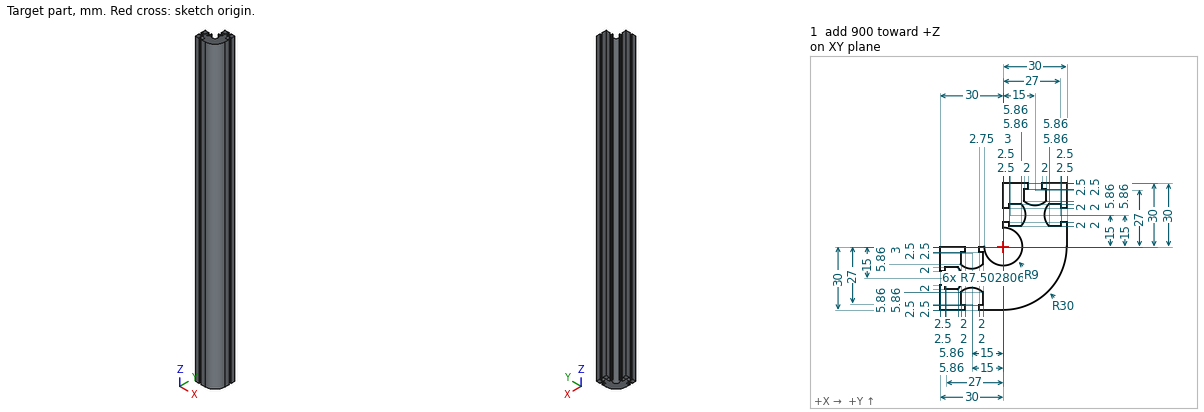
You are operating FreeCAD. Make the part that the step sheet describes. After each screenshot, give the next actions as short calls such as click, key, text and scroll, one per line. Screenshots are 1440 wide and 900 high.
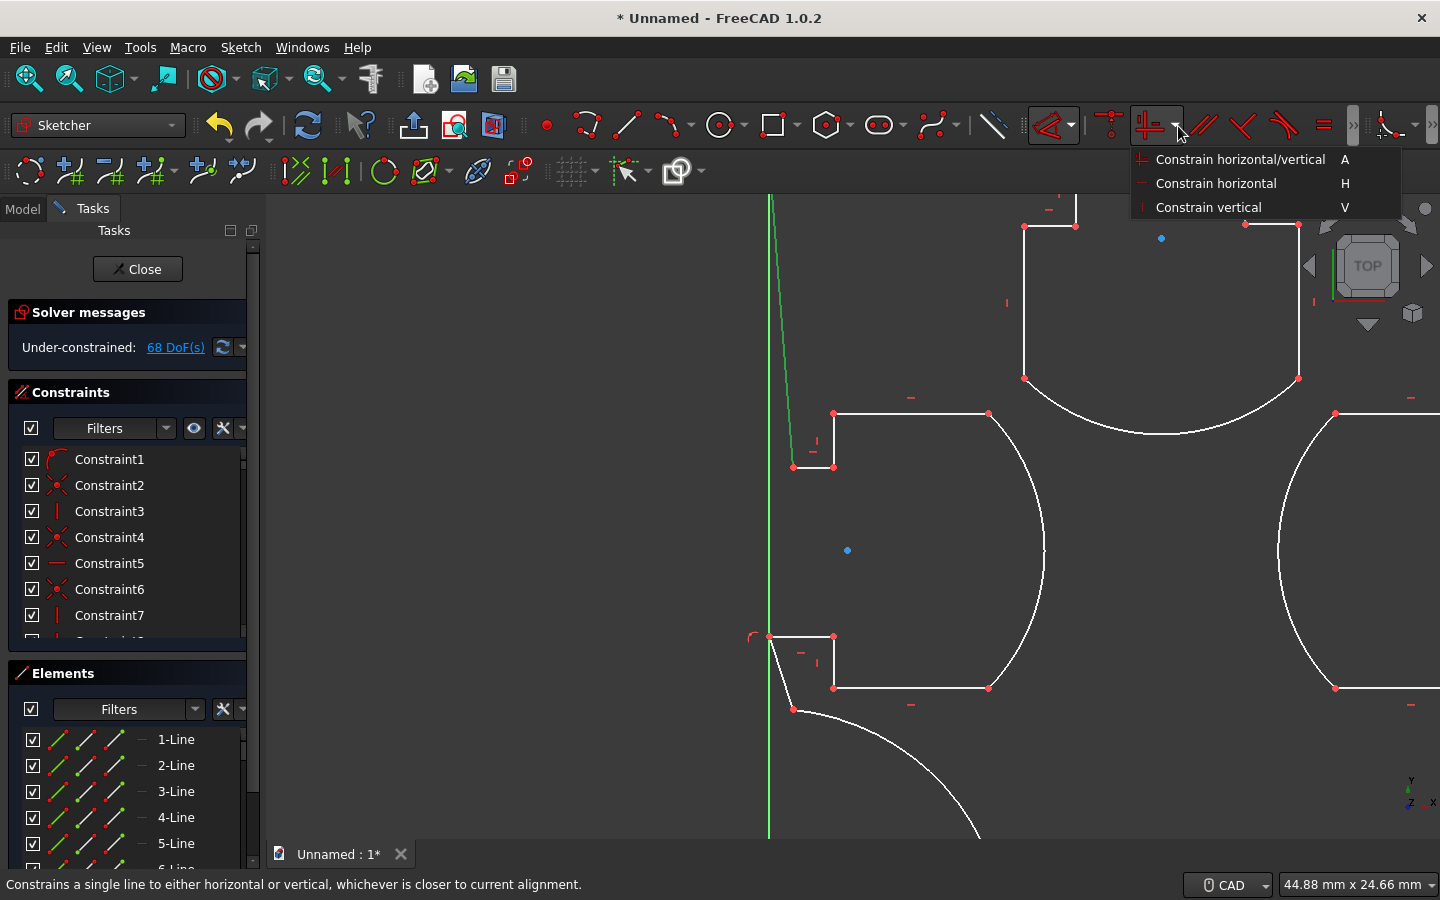
click(1266, 207)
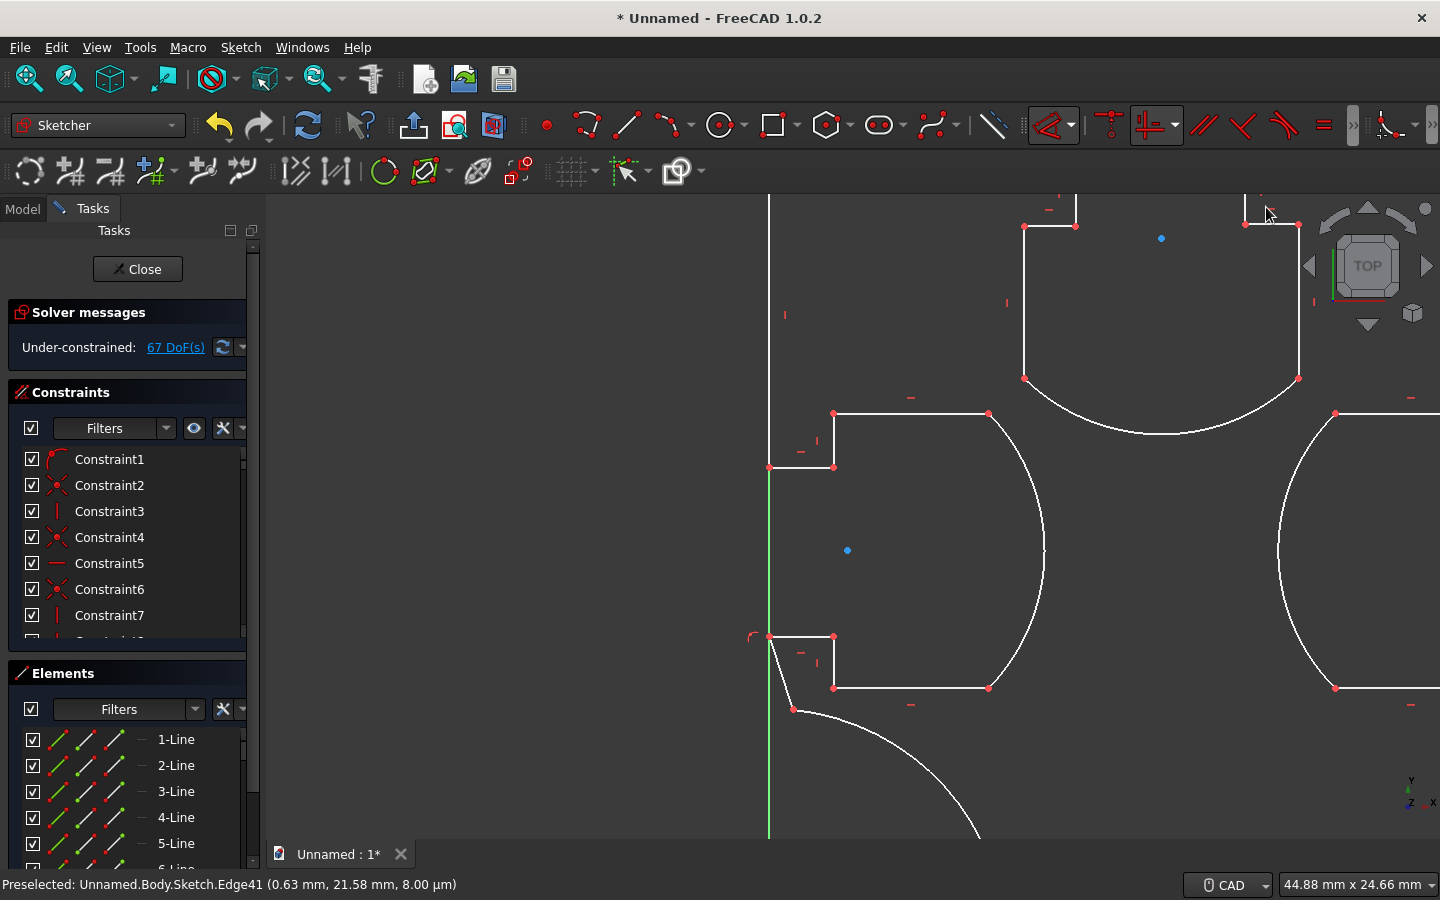
click(786, 688)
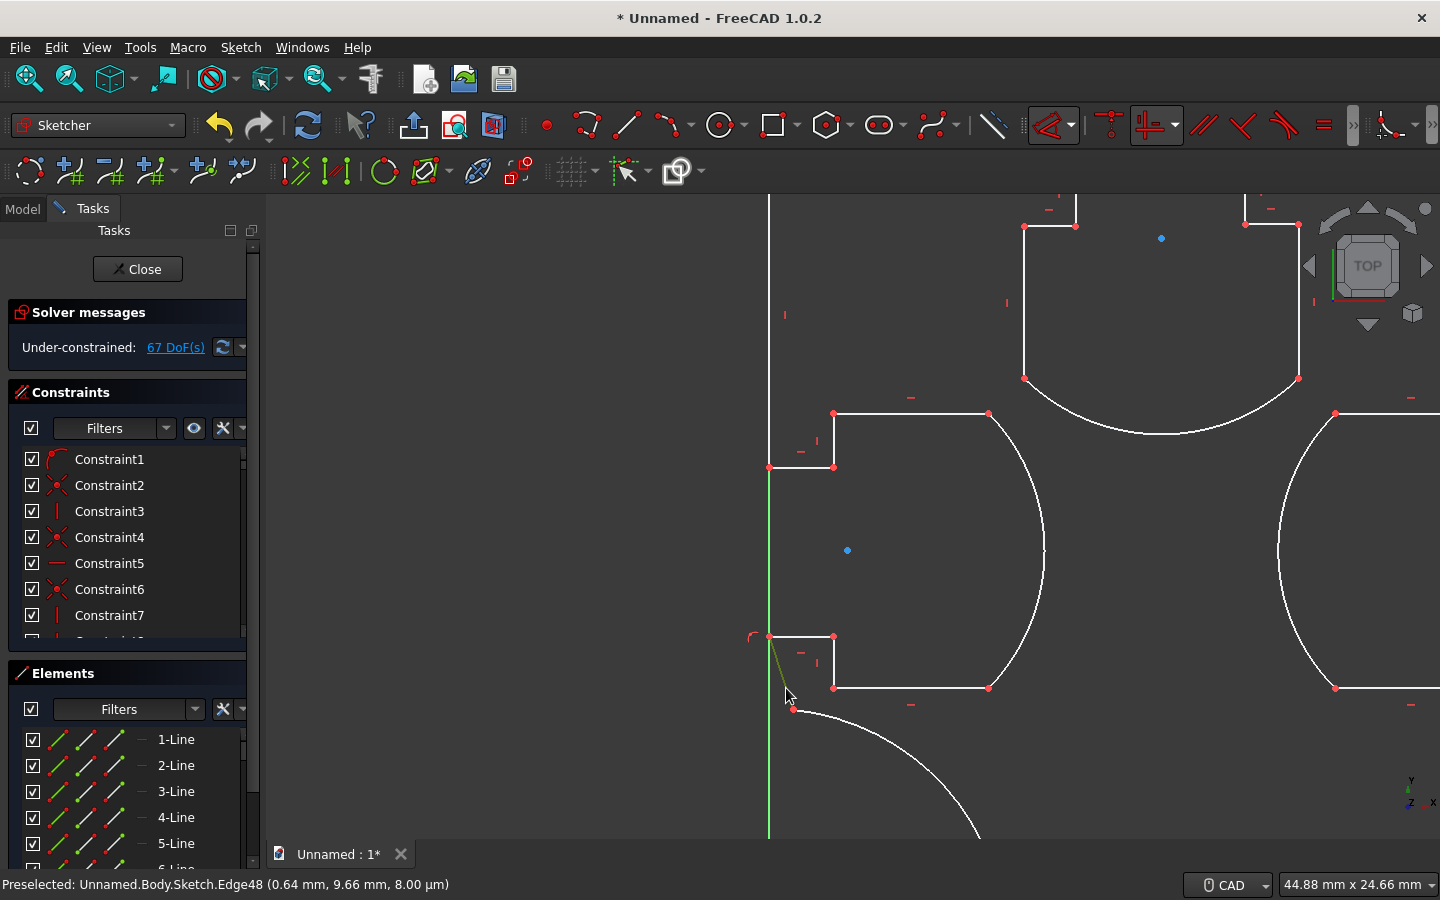
key(v)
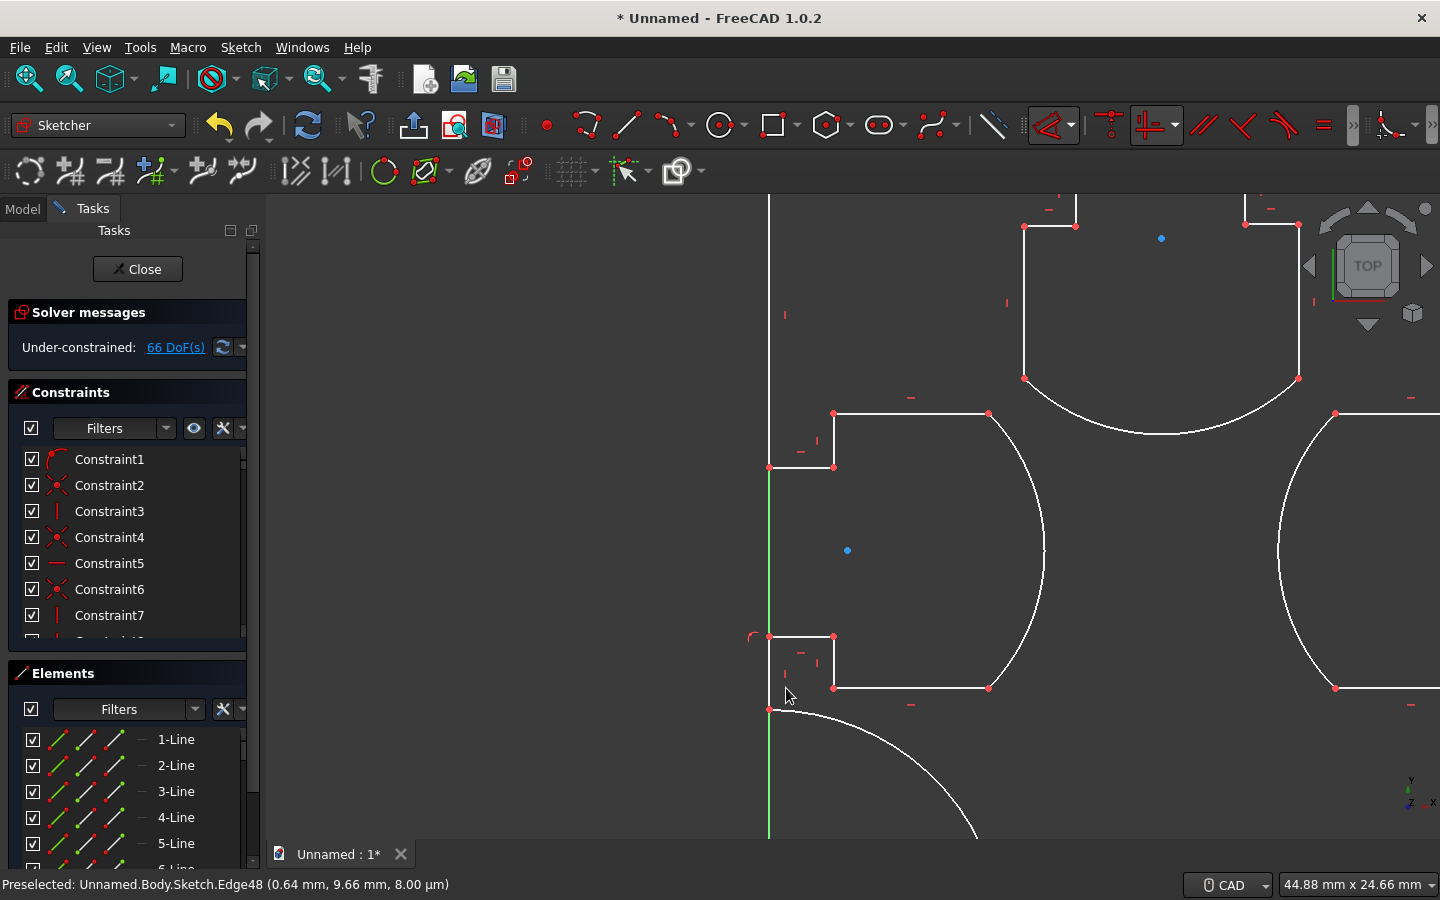
scroll(789, 377, down, 7)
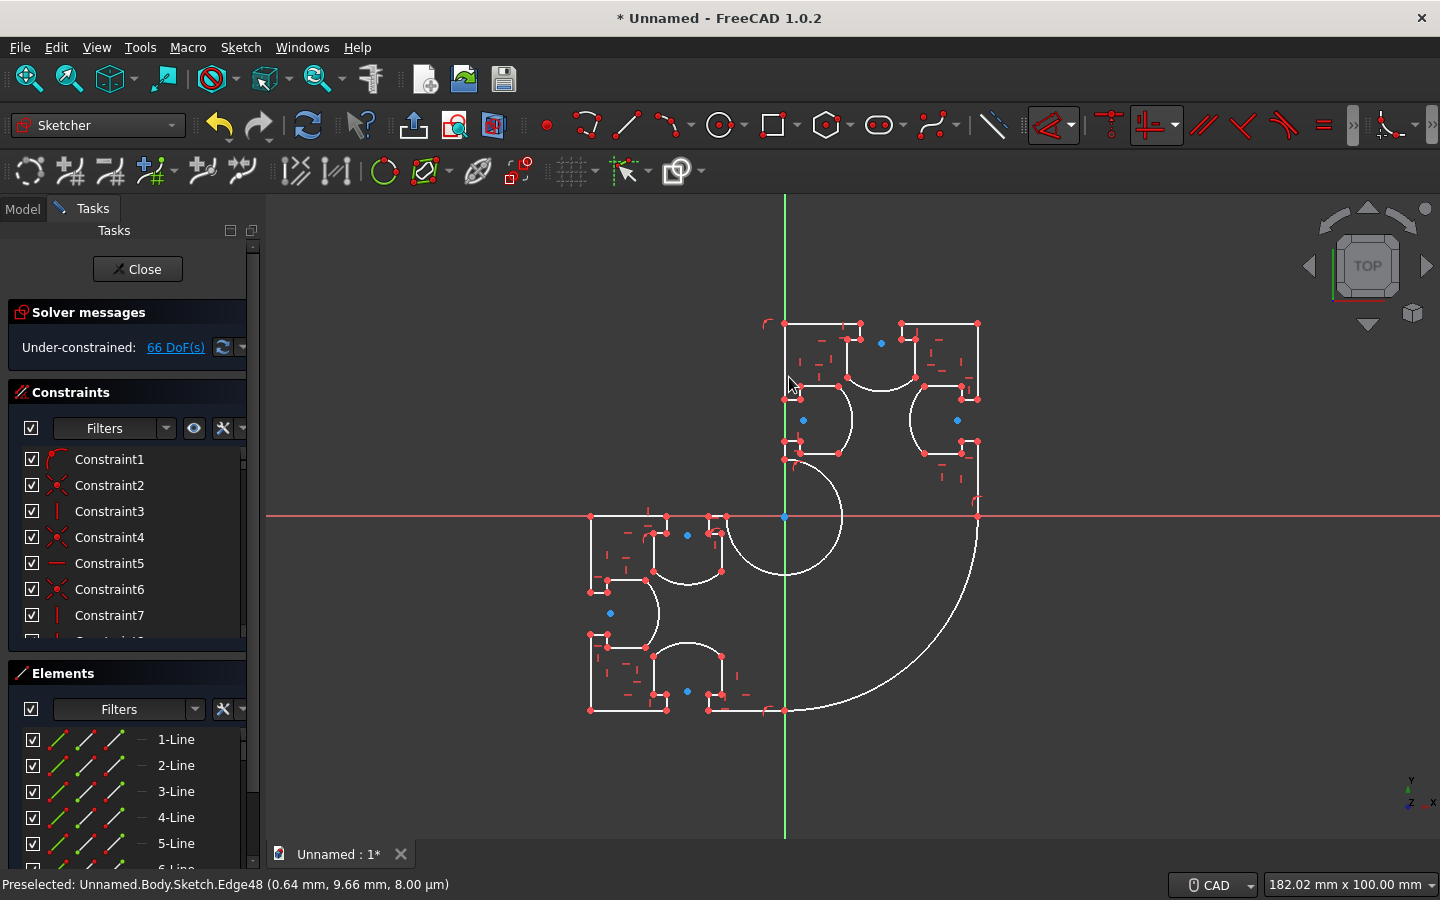
click(873, 690)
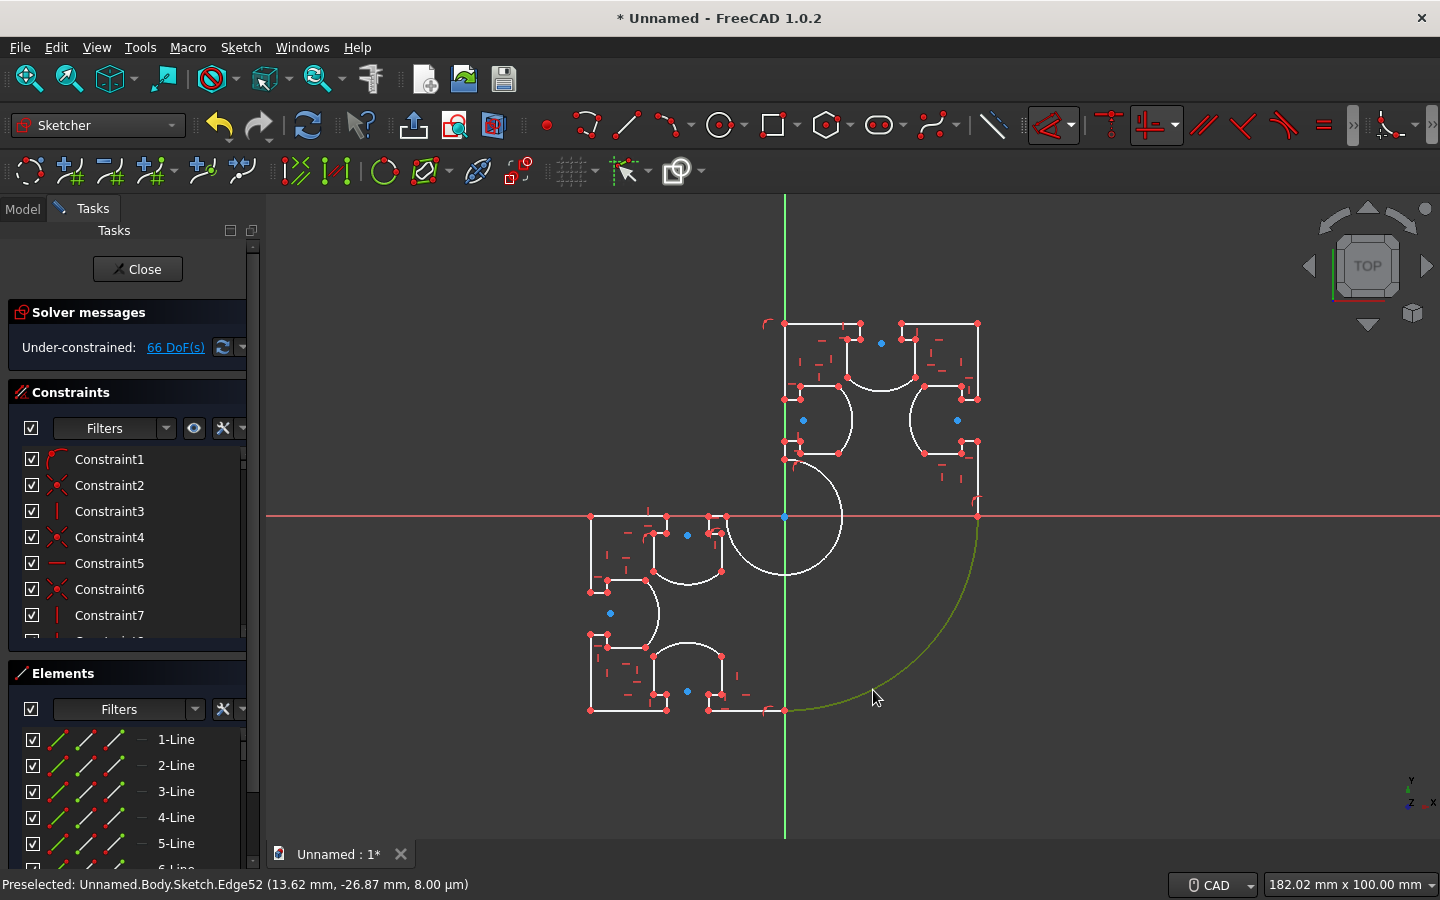
scroll(775, 574, up, 2)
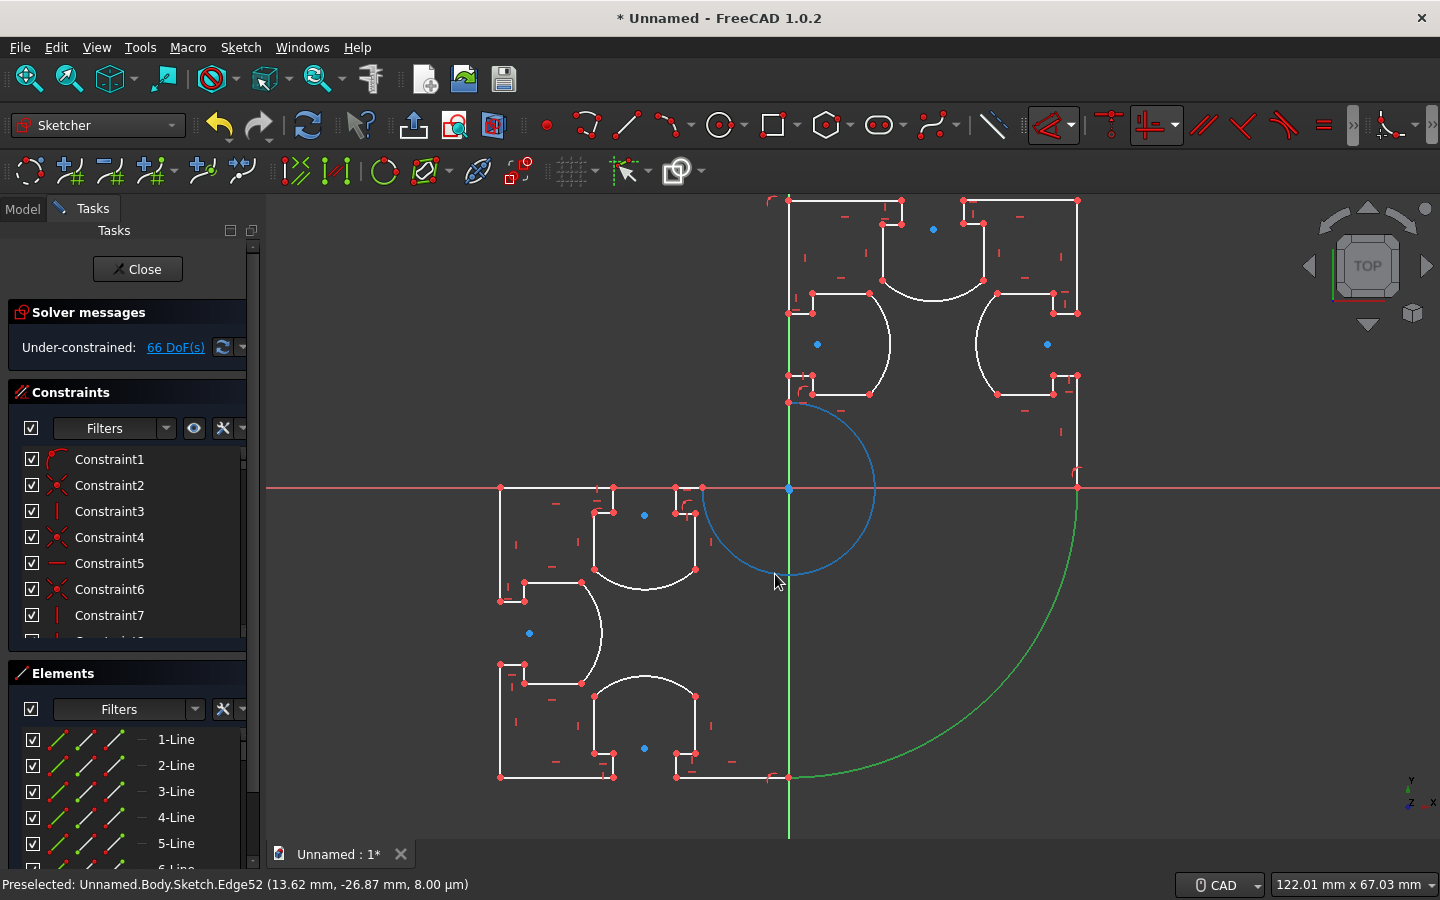
click(774, 574)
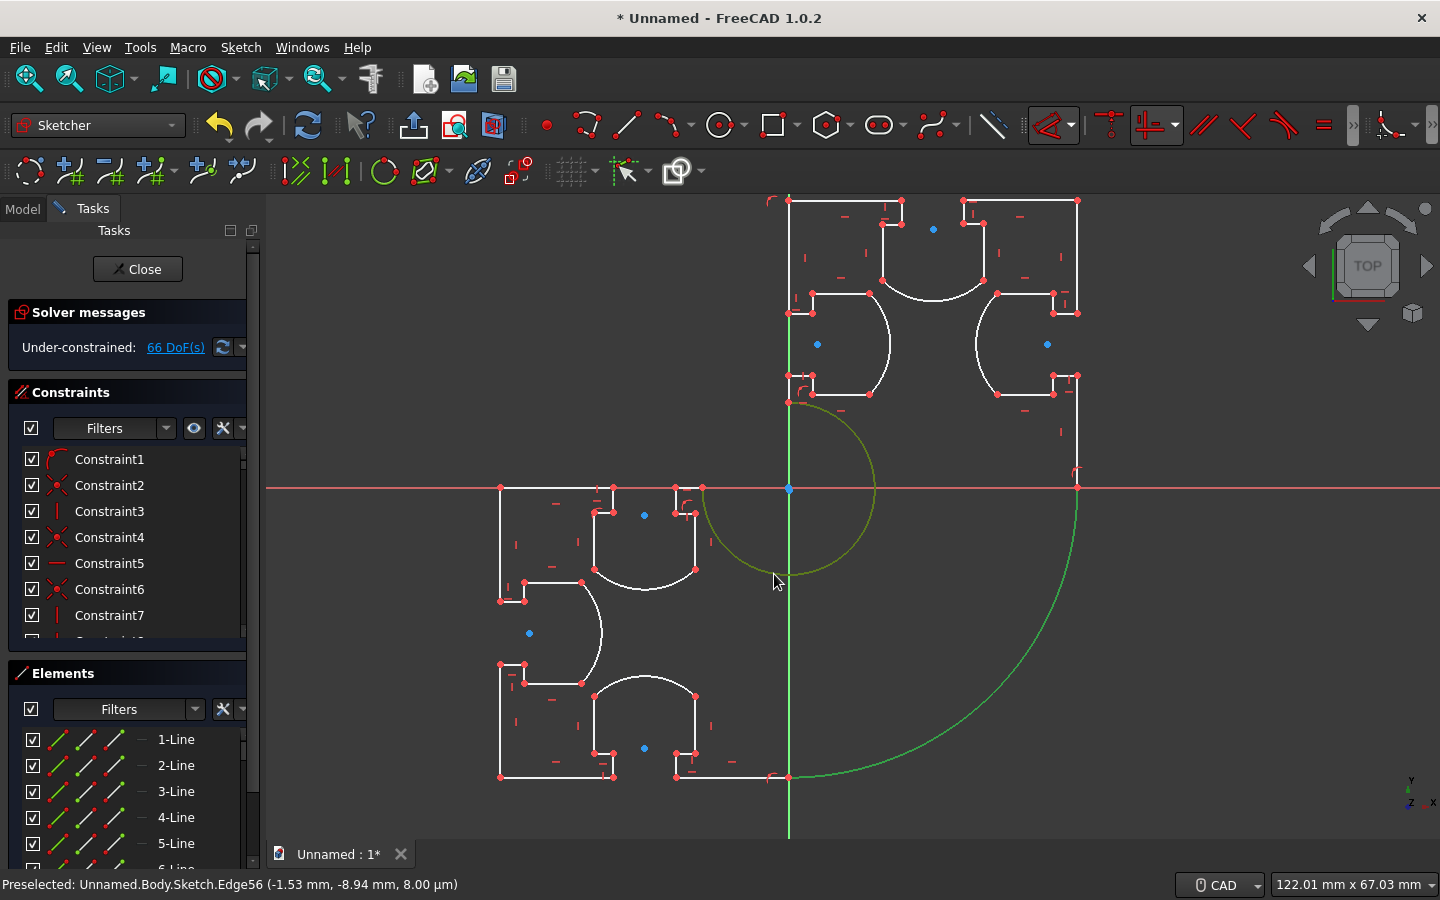
key(c)